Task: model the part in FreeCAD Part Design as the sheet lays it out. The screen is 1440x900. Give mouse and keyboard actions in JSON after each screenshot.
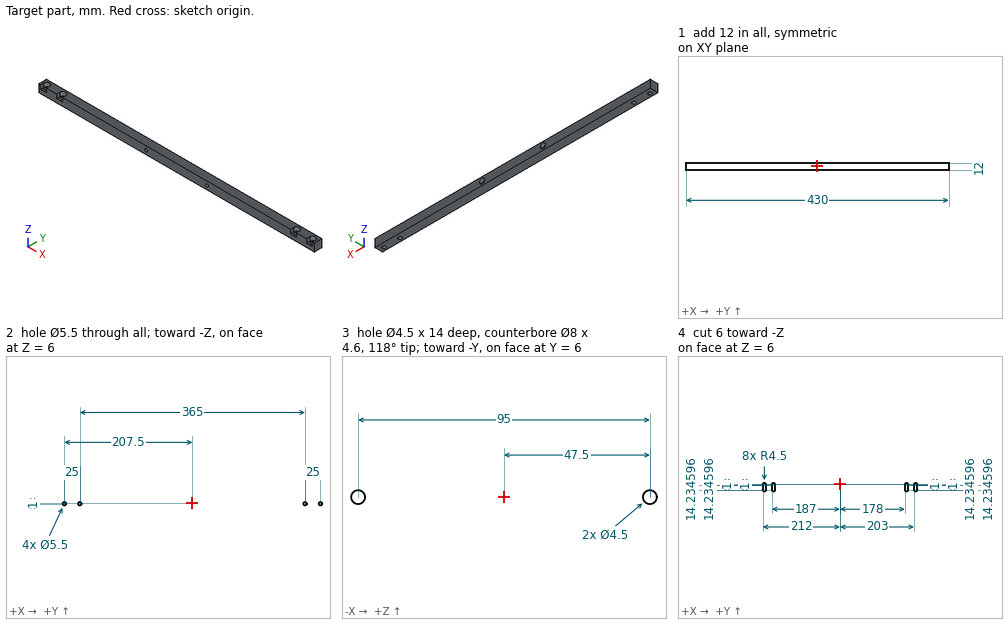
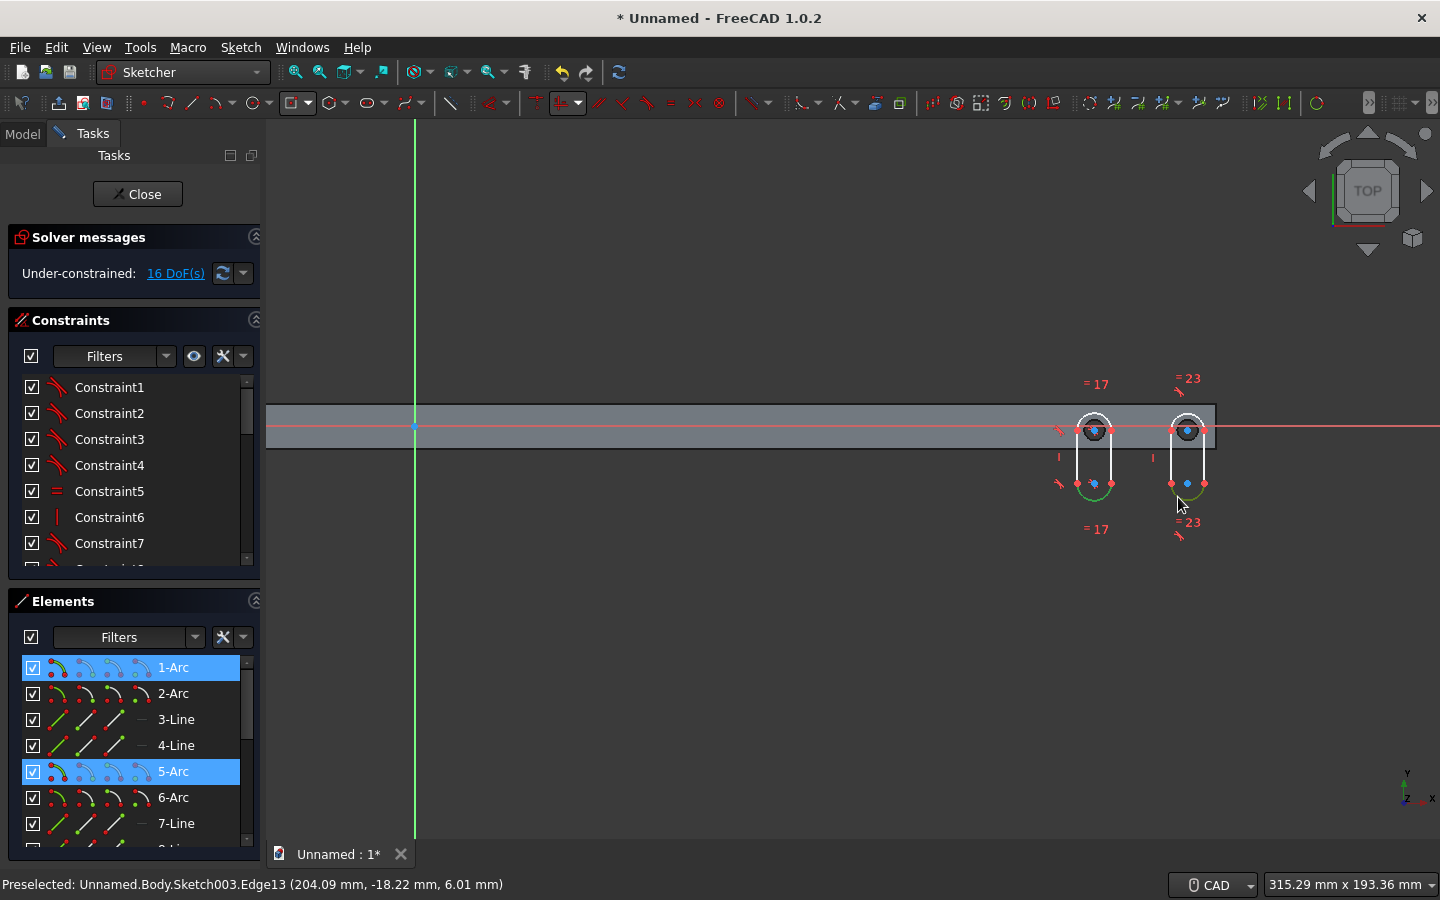
{"action": "left_click", "coordinate": [672, 104]}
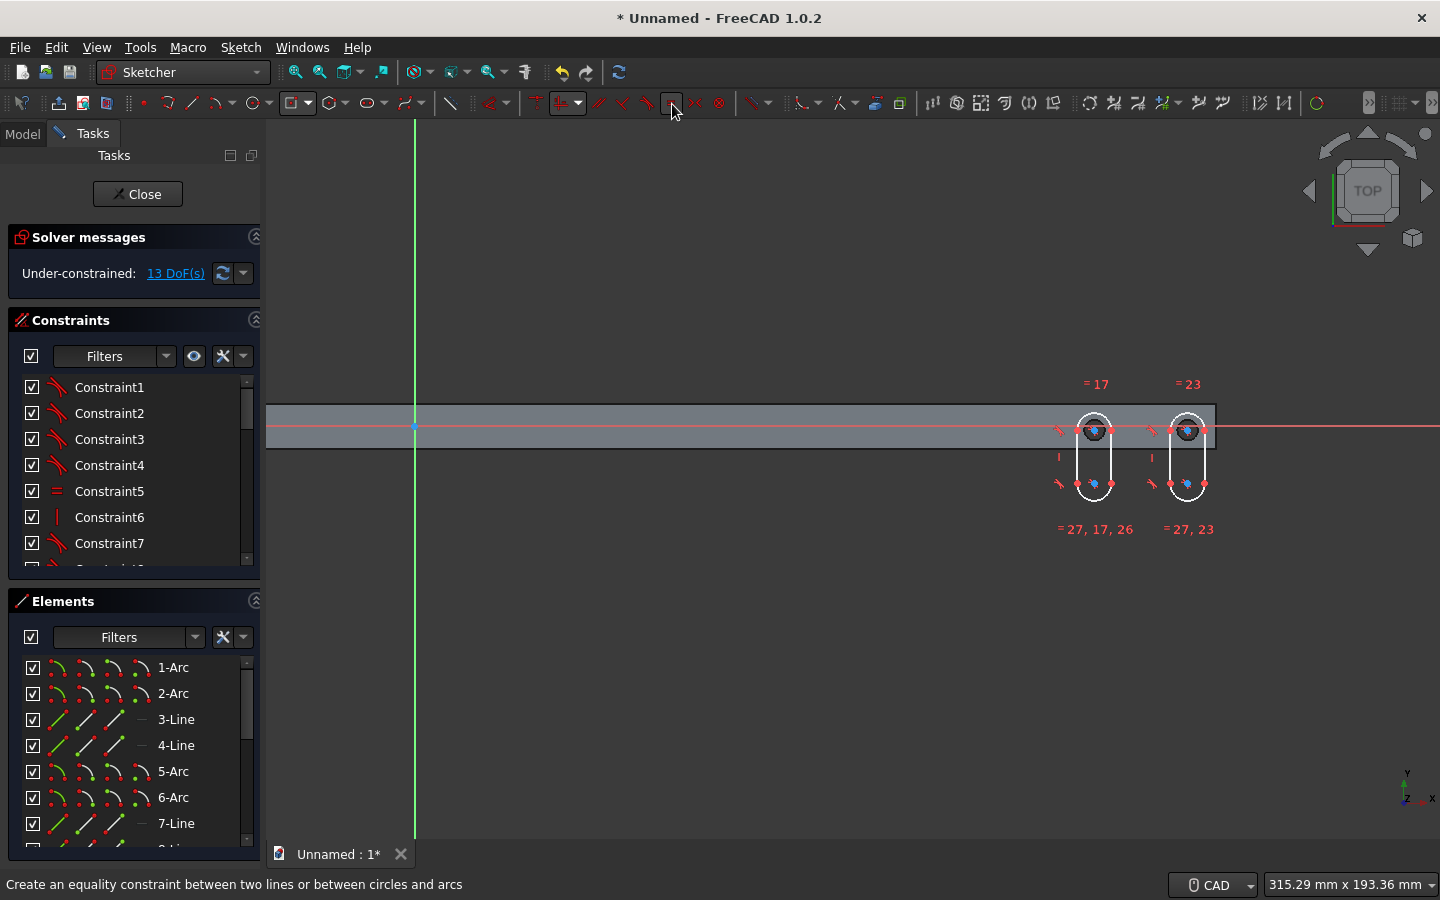
{"action": "left_click", "coordinate": [490, 104]}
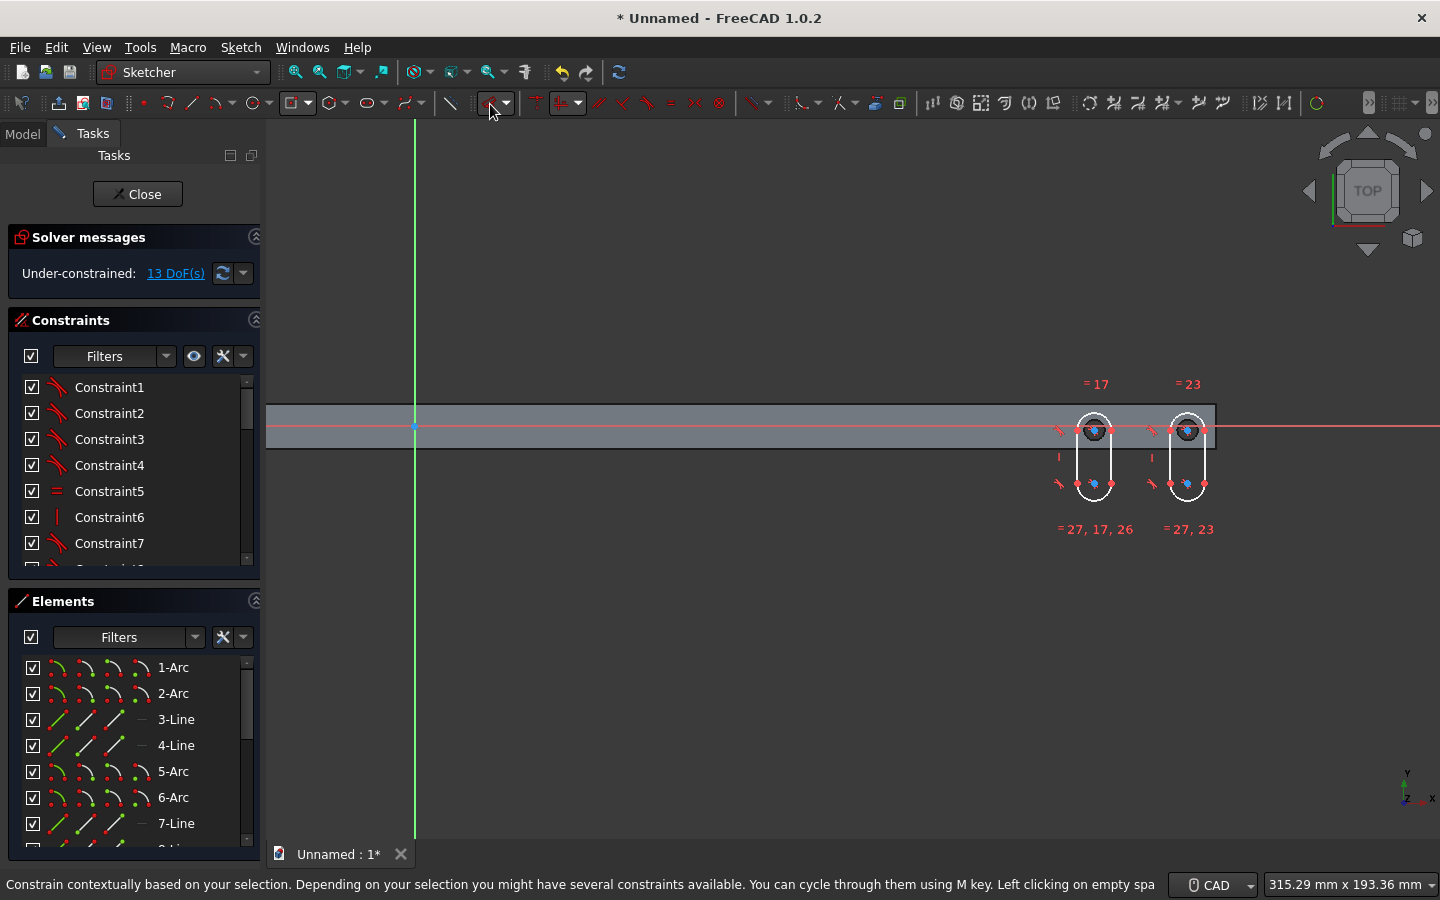
{"action": "scroll", "coordinate": [1086, 497], "scroll_direction": "down", "scroll_amount": 4}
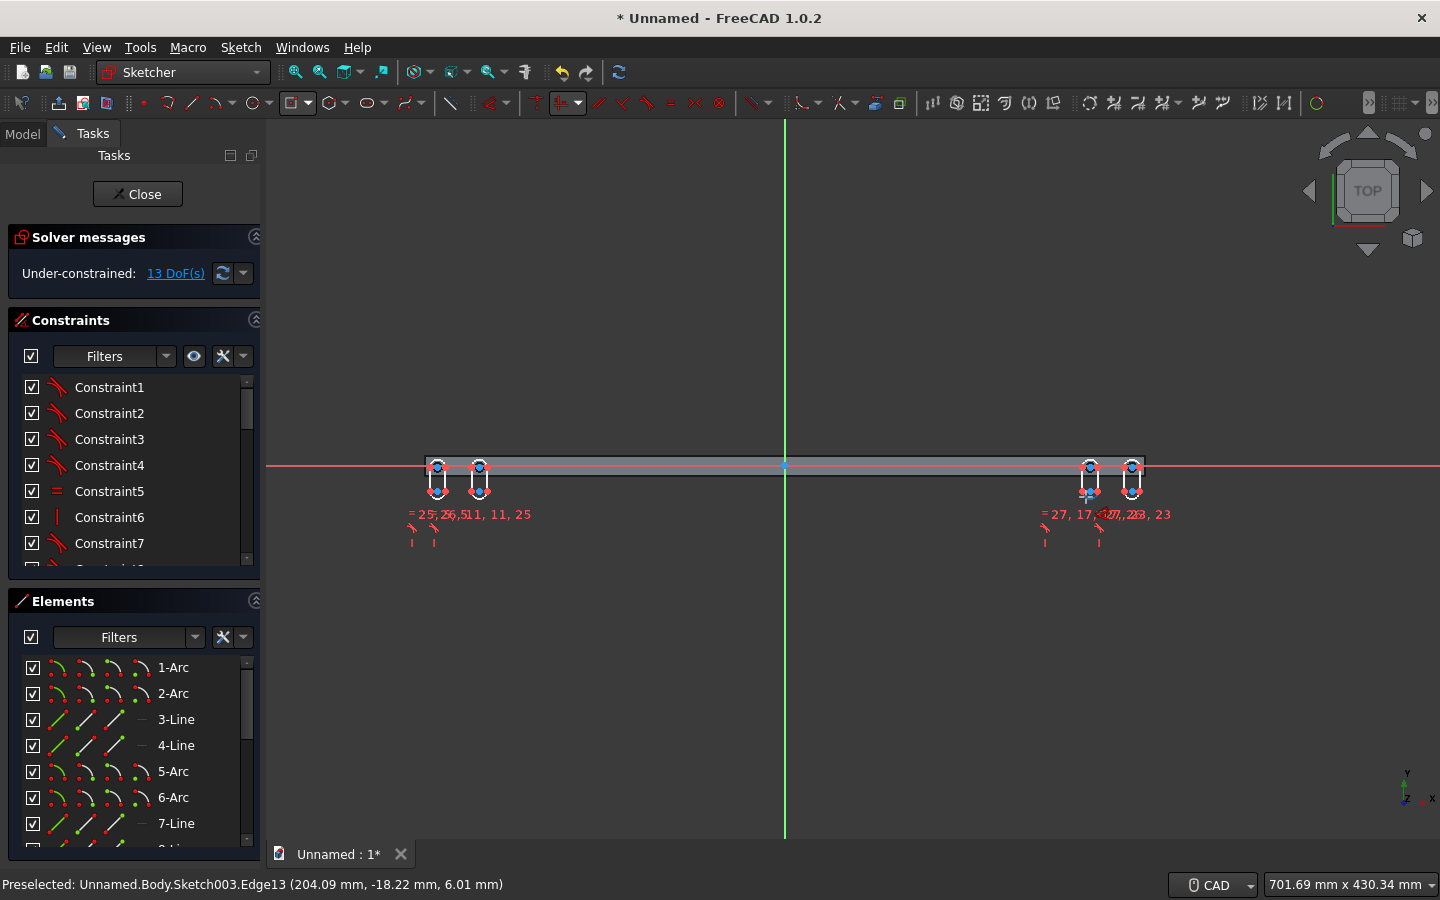
{"action": "scroll", "coordinate": [433, 497], "scroll_direction": "up", "scroll_amount": 9}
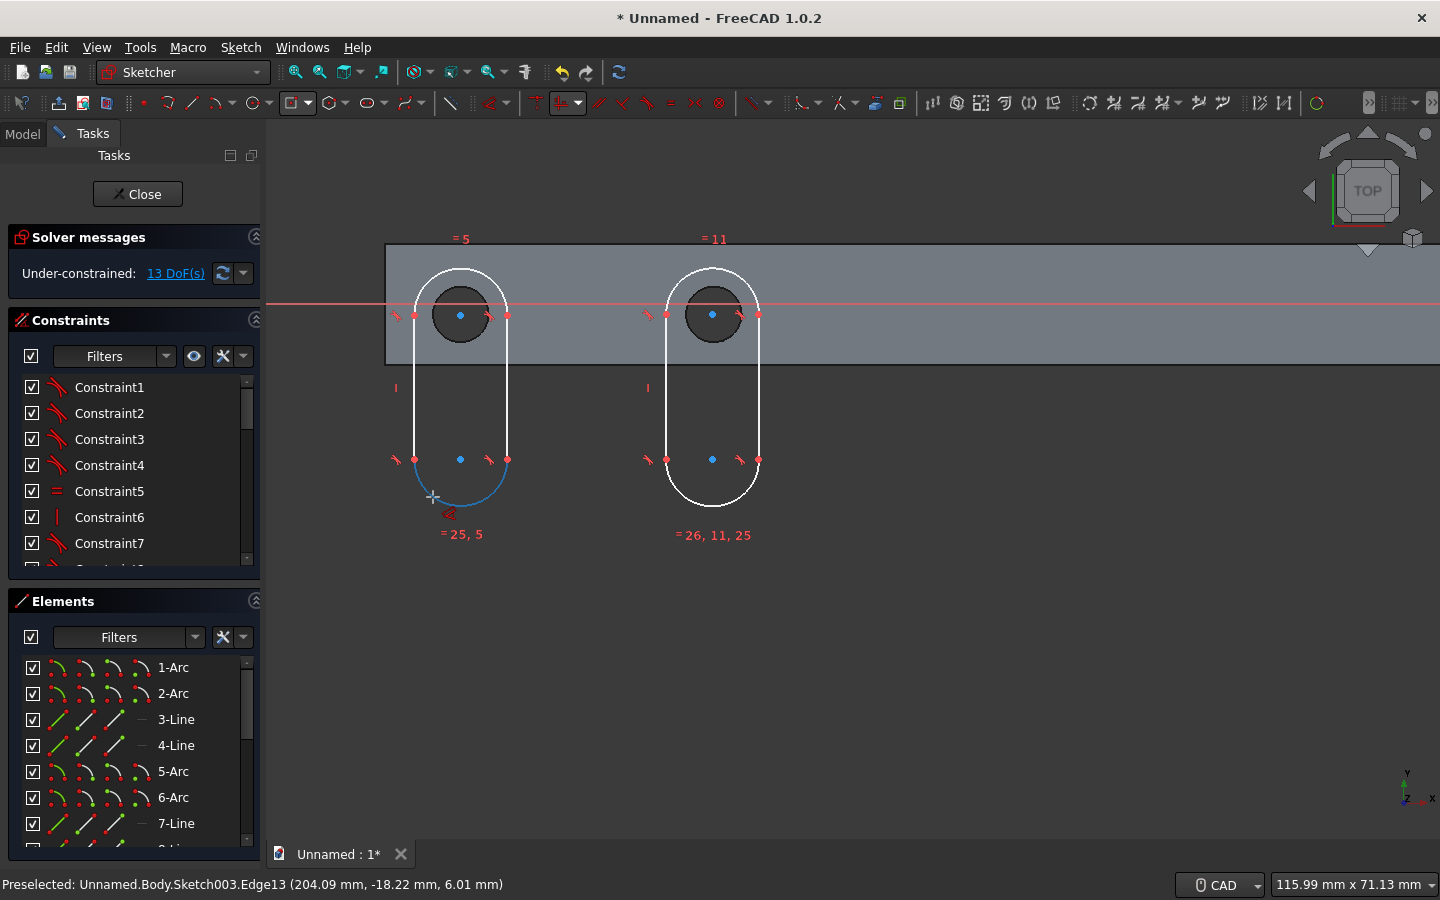
{"action": "left_click", "coordinate": [434, 497]}
{"action": "left_click", "coordinate": [415, 523]}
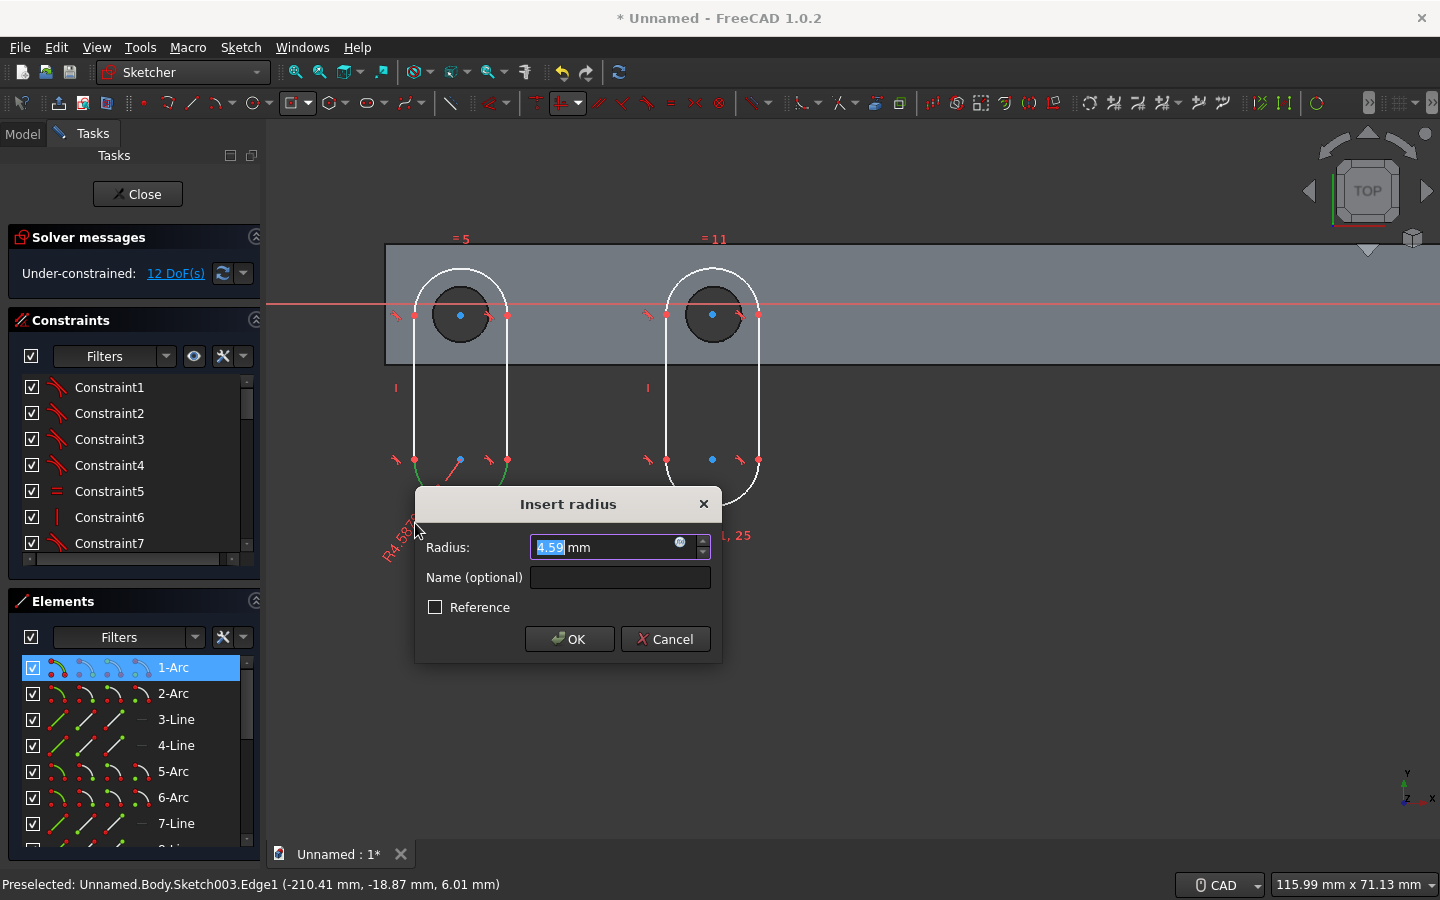
{"action": "type", "text": "4.5"}
{"action": "key", "text": "Return"}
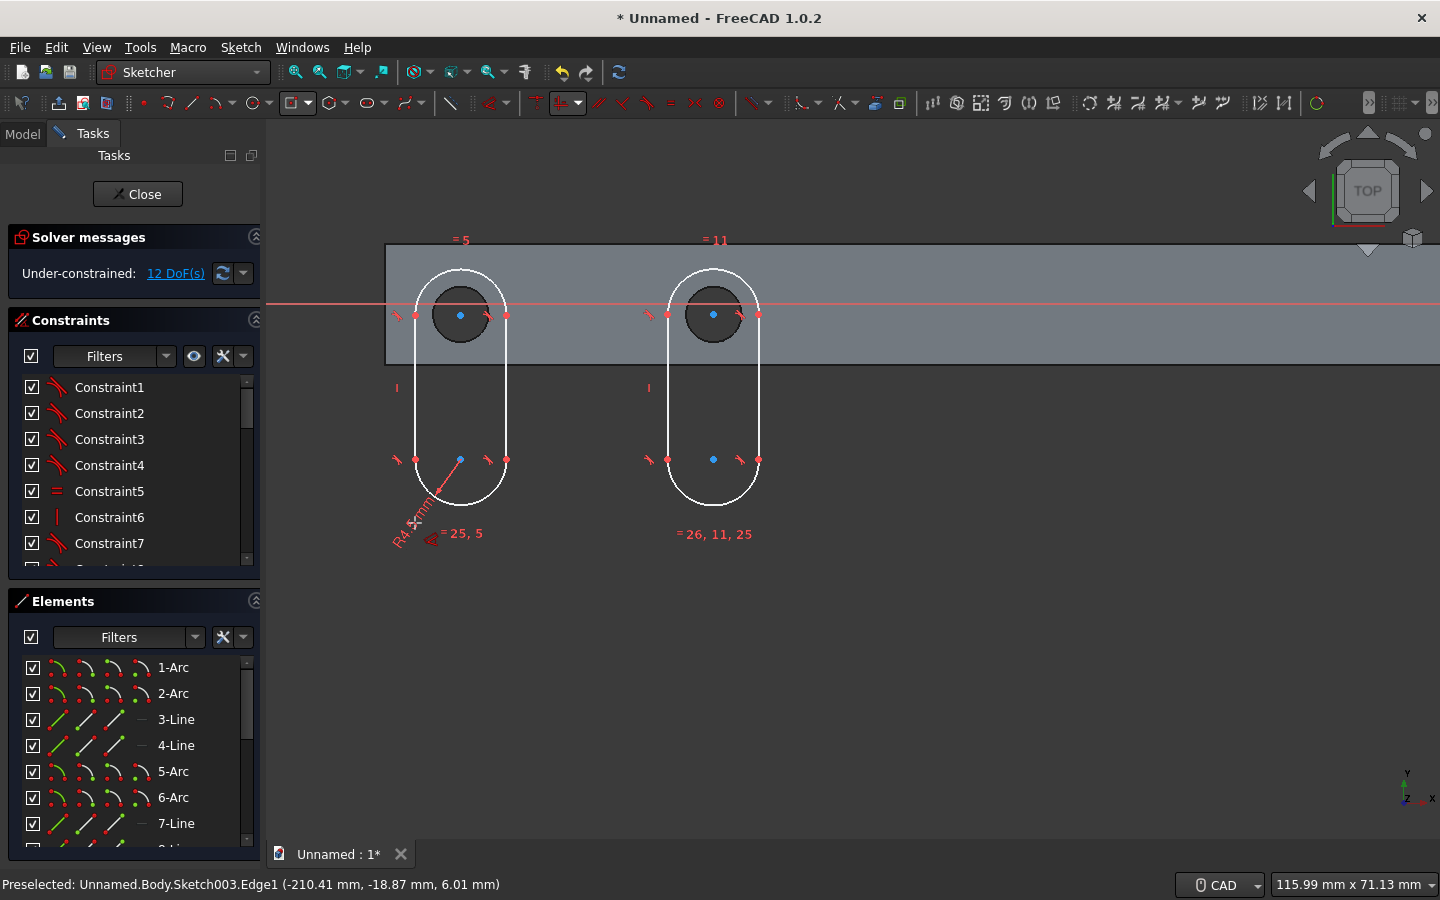
{"action": "scroll", "coordinate": [506, 315], "scroll_direction": "up", "scroll_amount": 7}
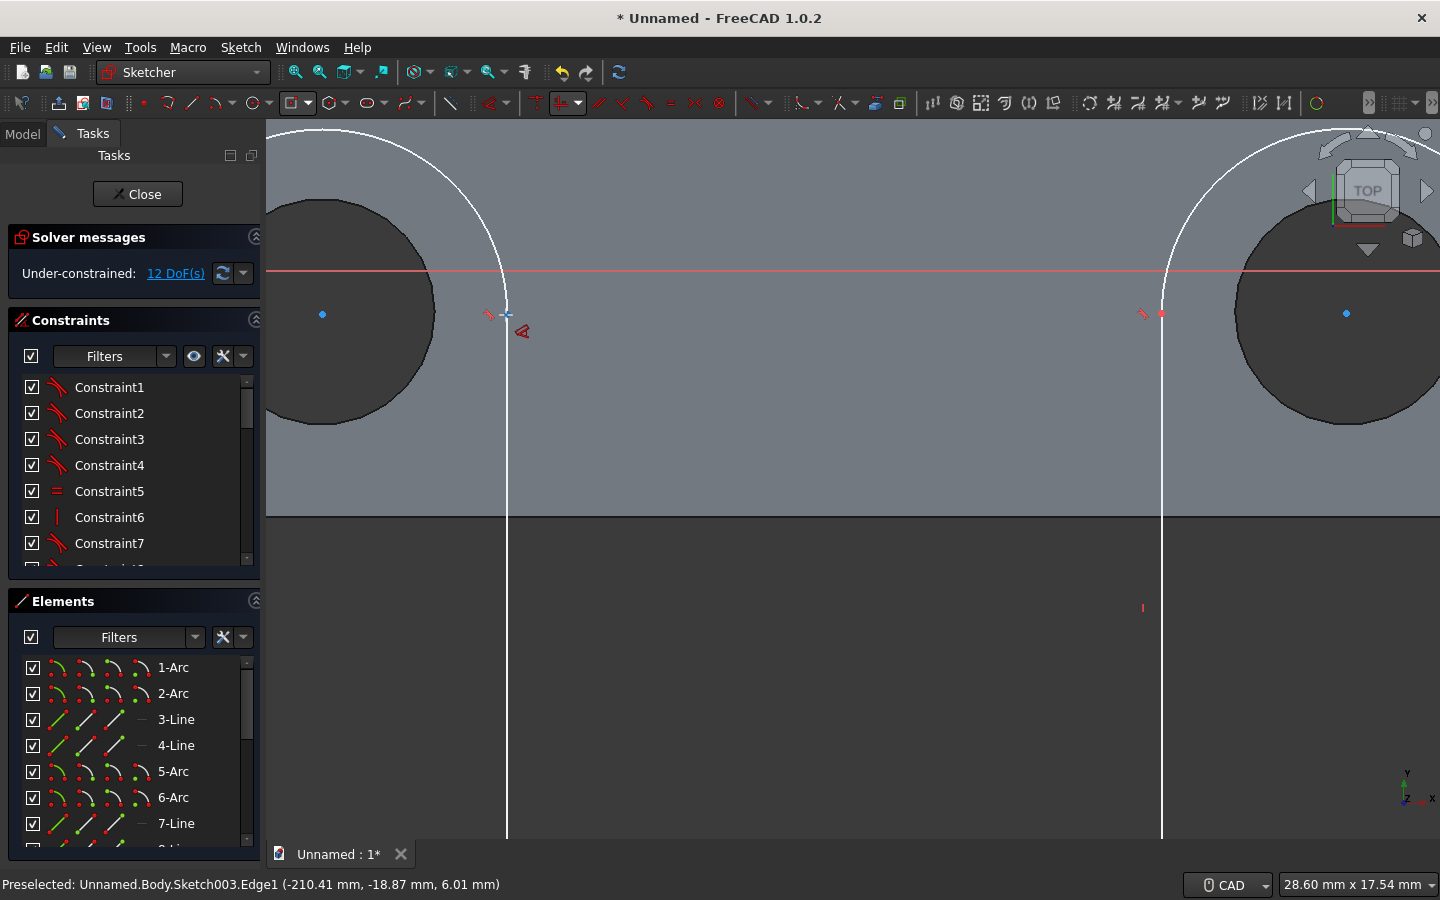
{"action": "left_click", "coordinate": [507, 314]}
{"action": "left_click", "coordinate": [473, 292]}